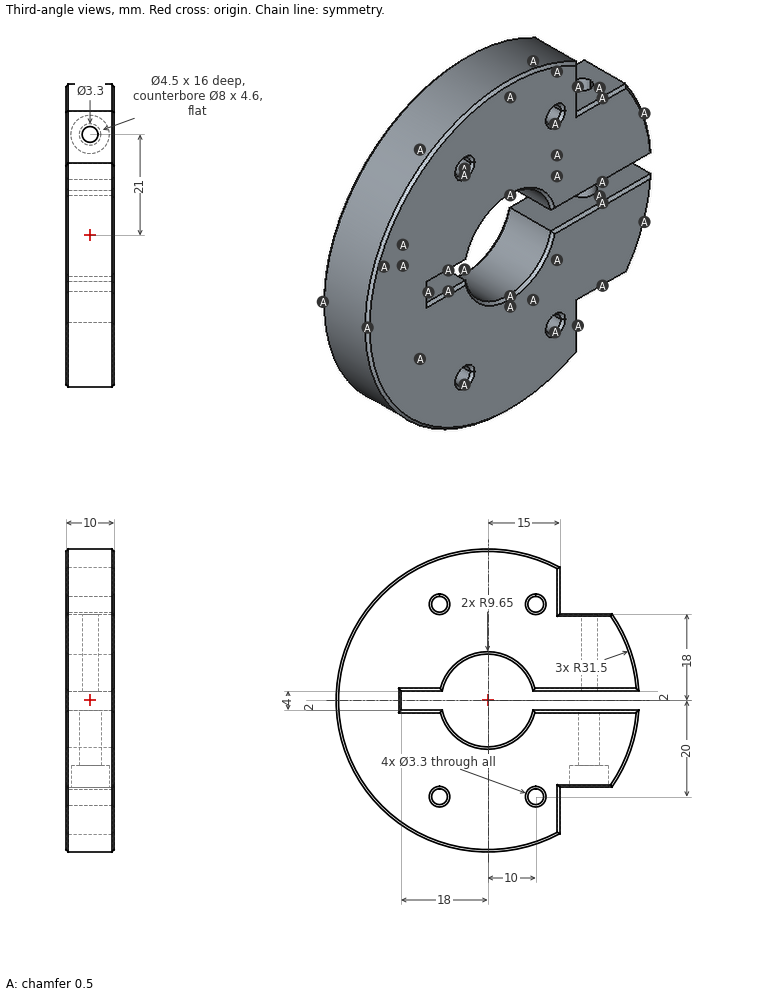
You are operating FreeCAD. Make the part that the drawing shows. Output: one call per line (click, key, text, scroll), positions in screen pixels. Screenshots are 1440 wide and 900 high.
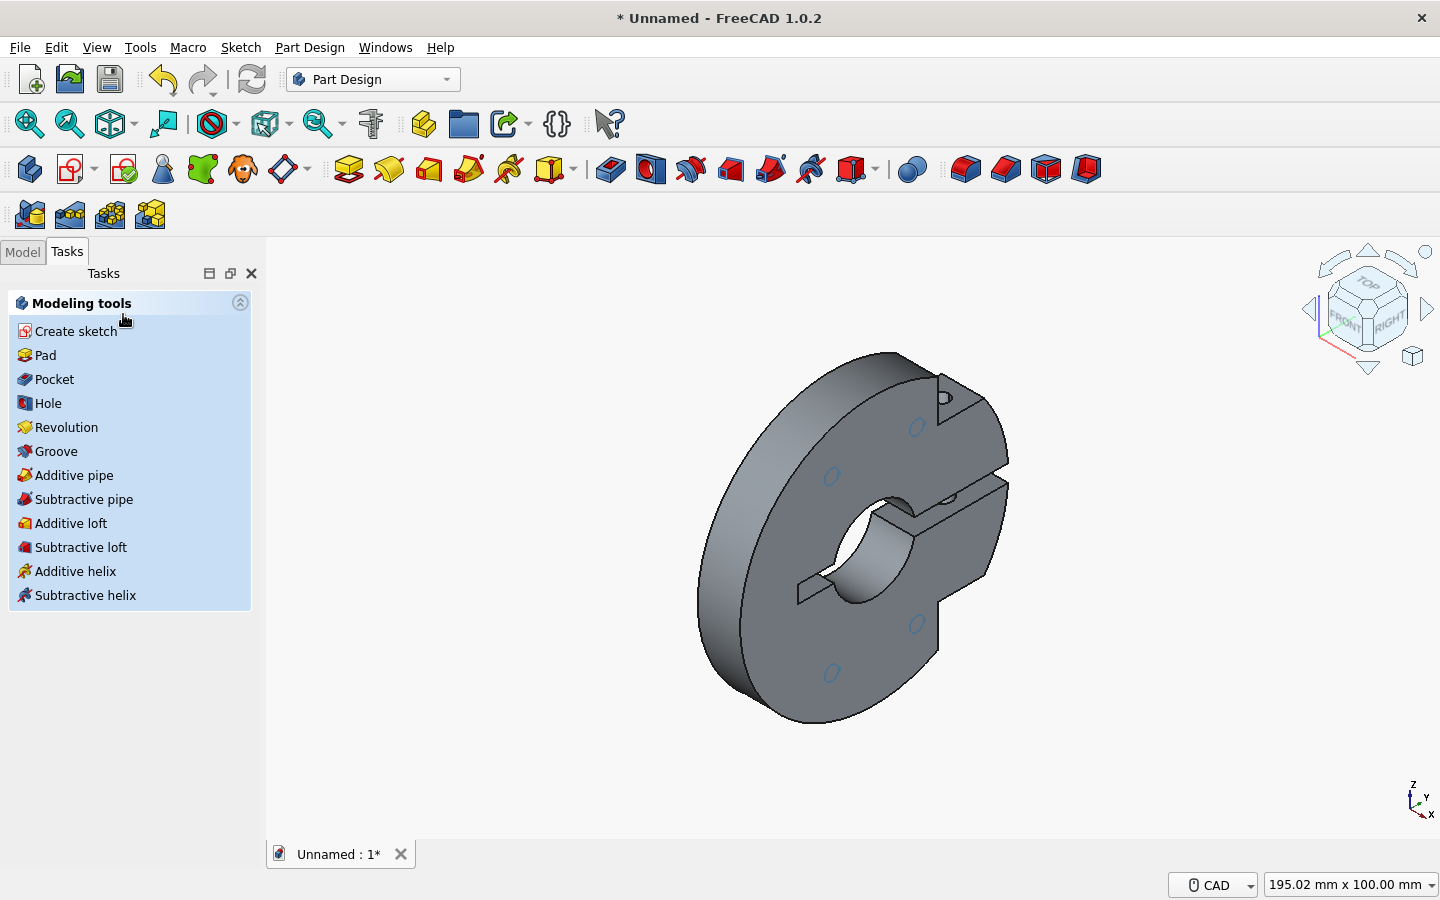
click(652, 170)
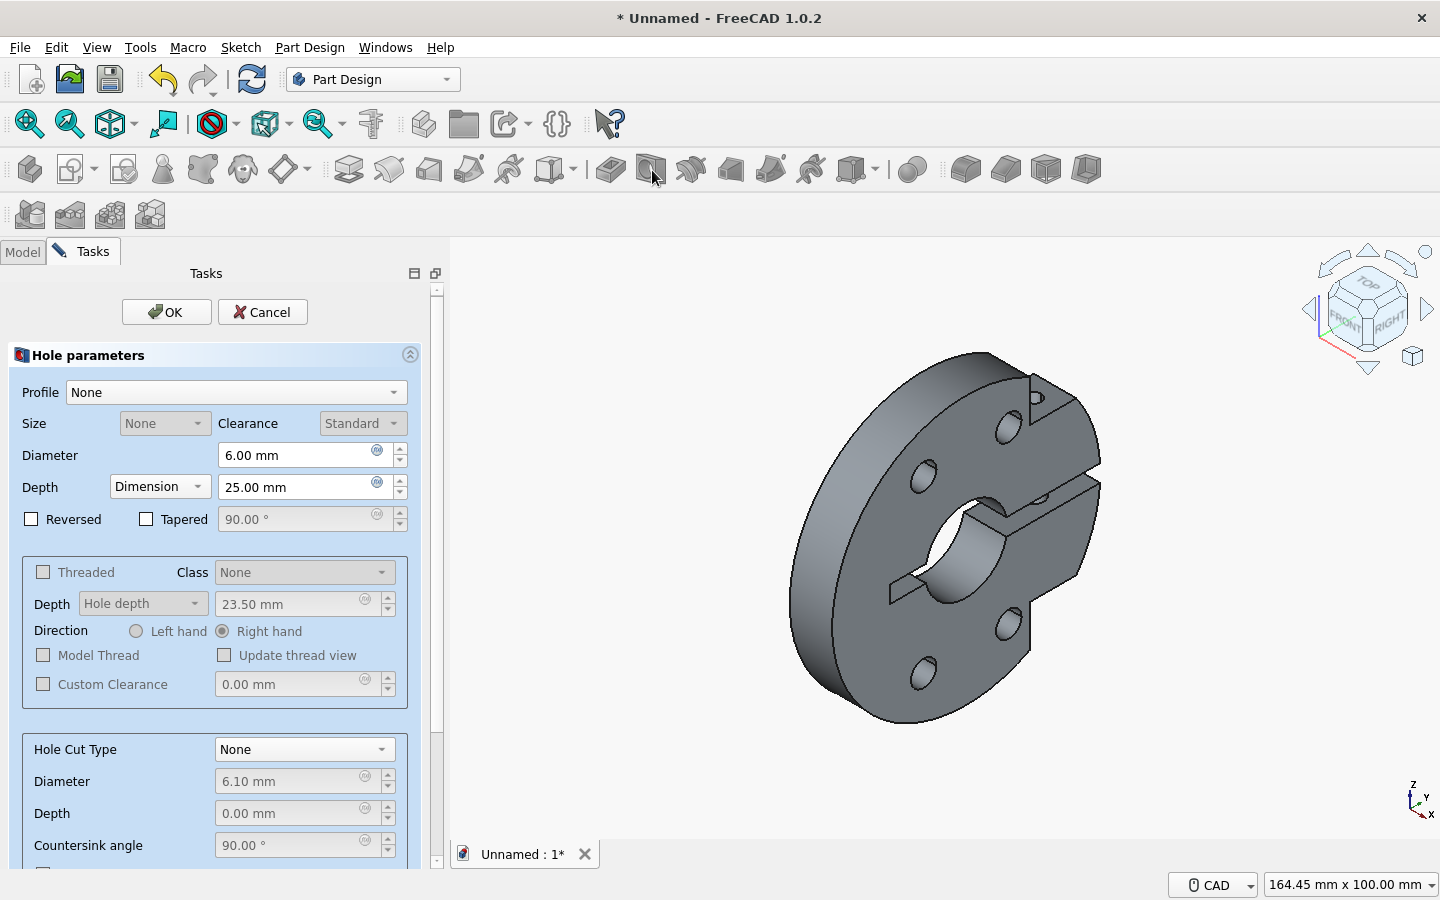
triple_click(305, 455)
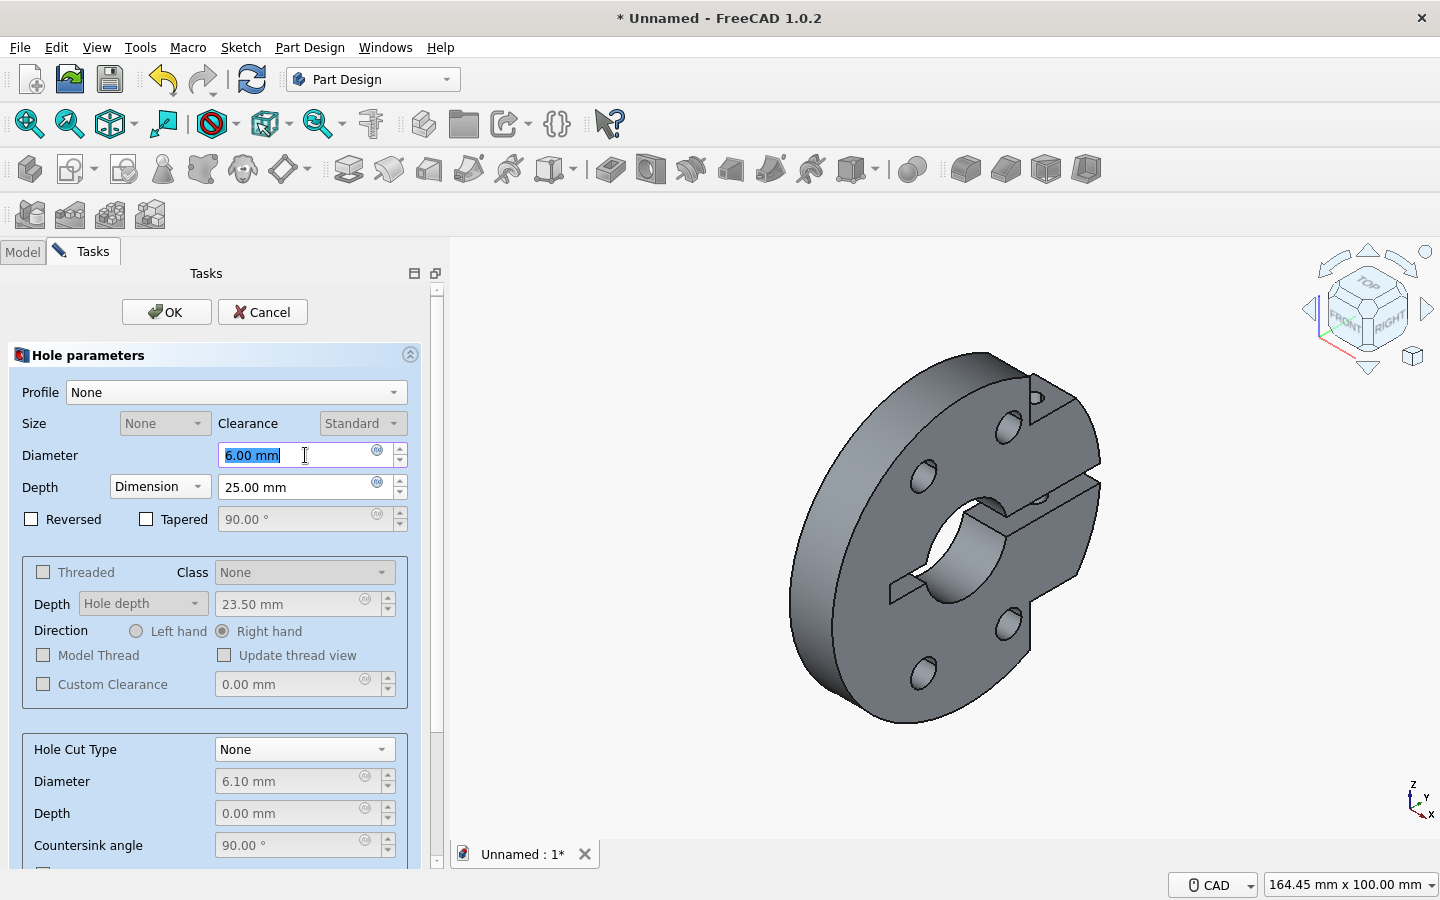
text(3.3)
key(Tab)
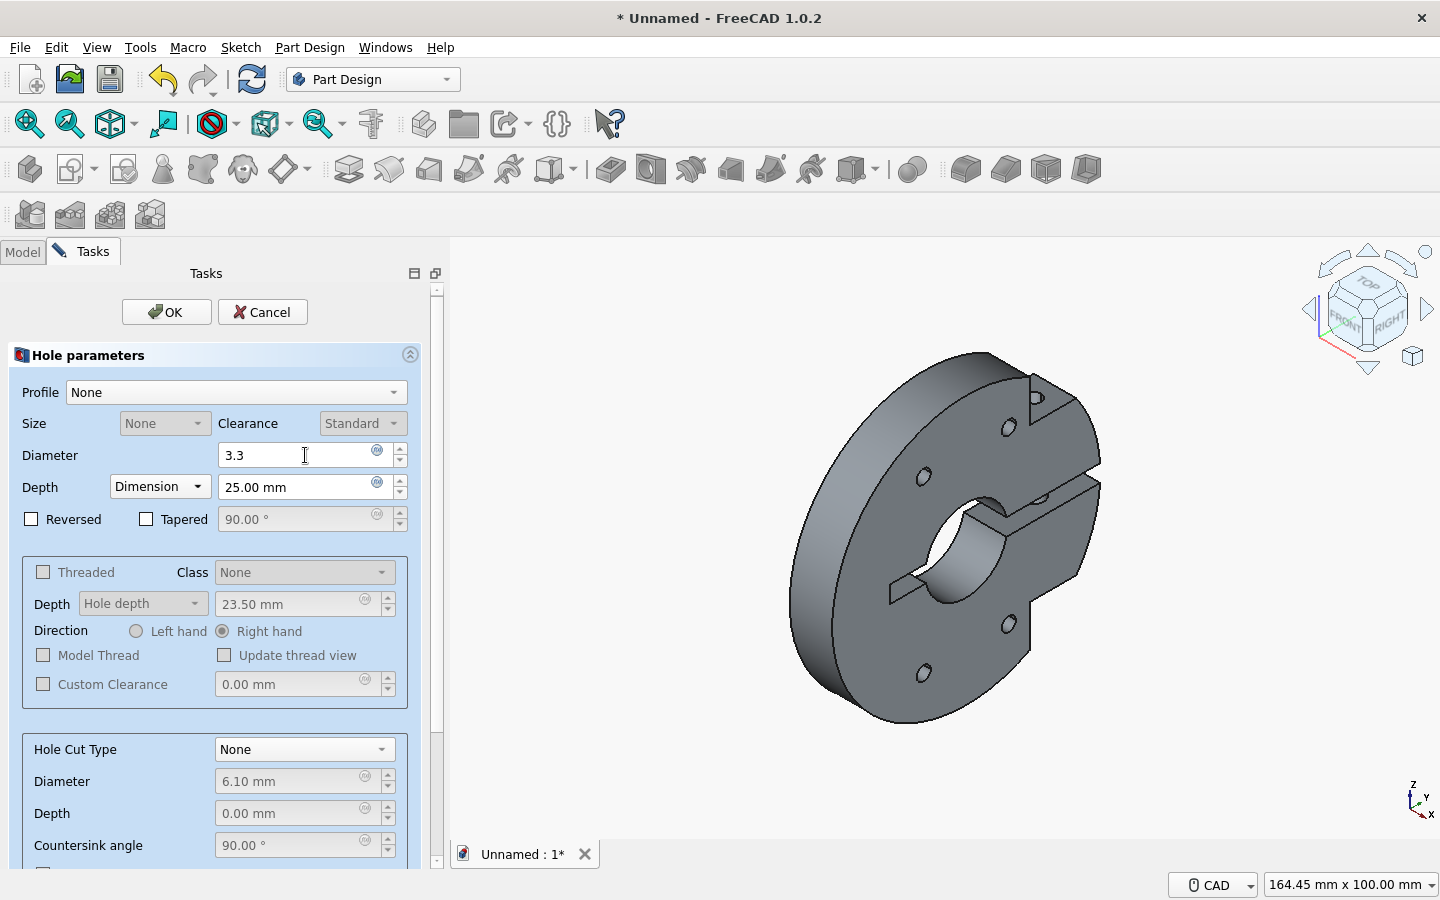
click(161, 486)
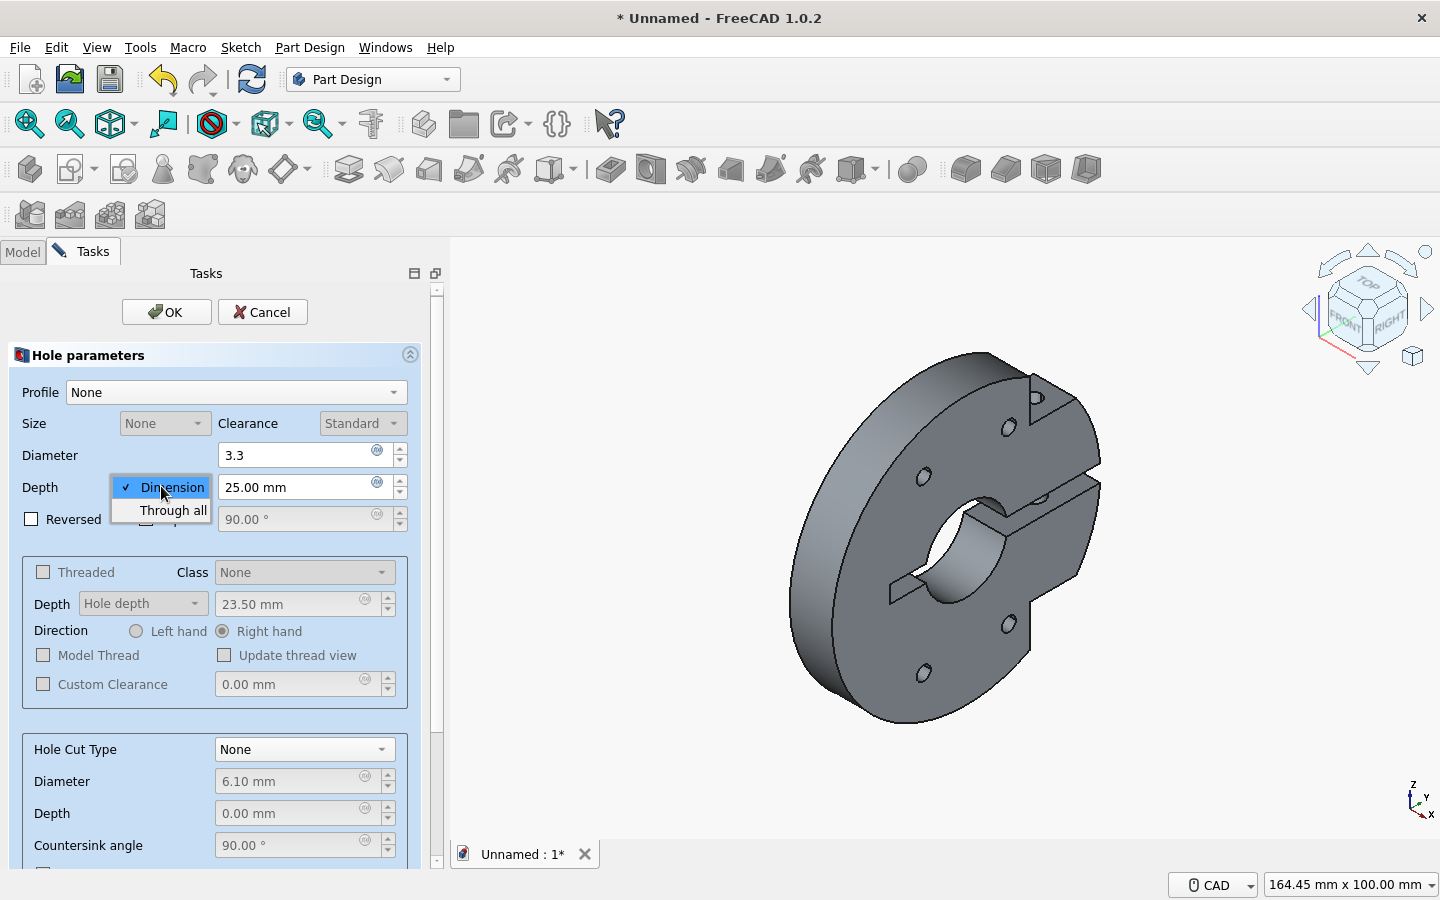
click(160, 510)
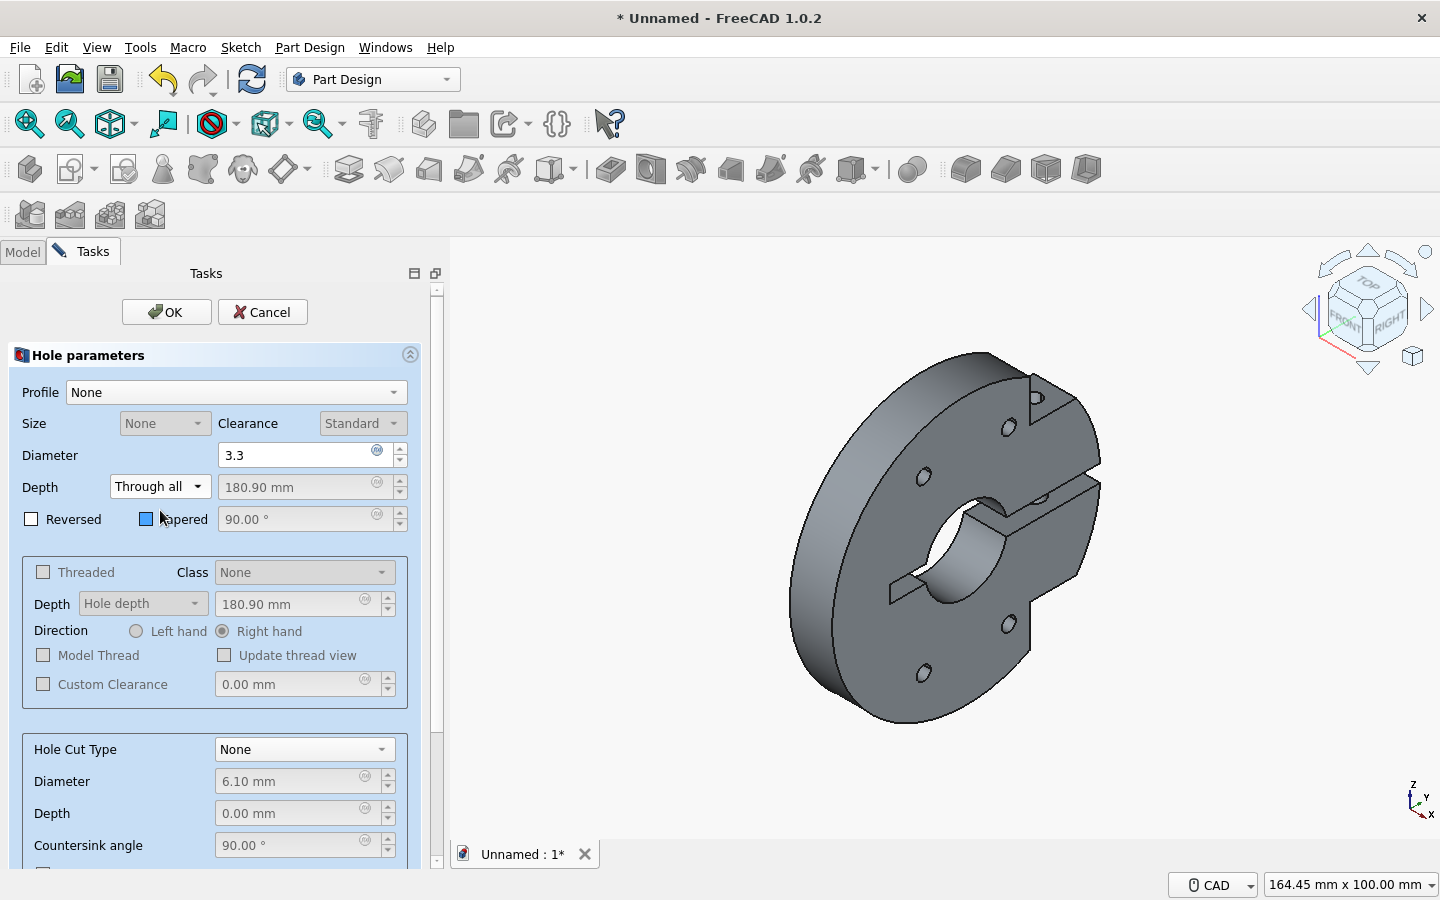
click(167, 312)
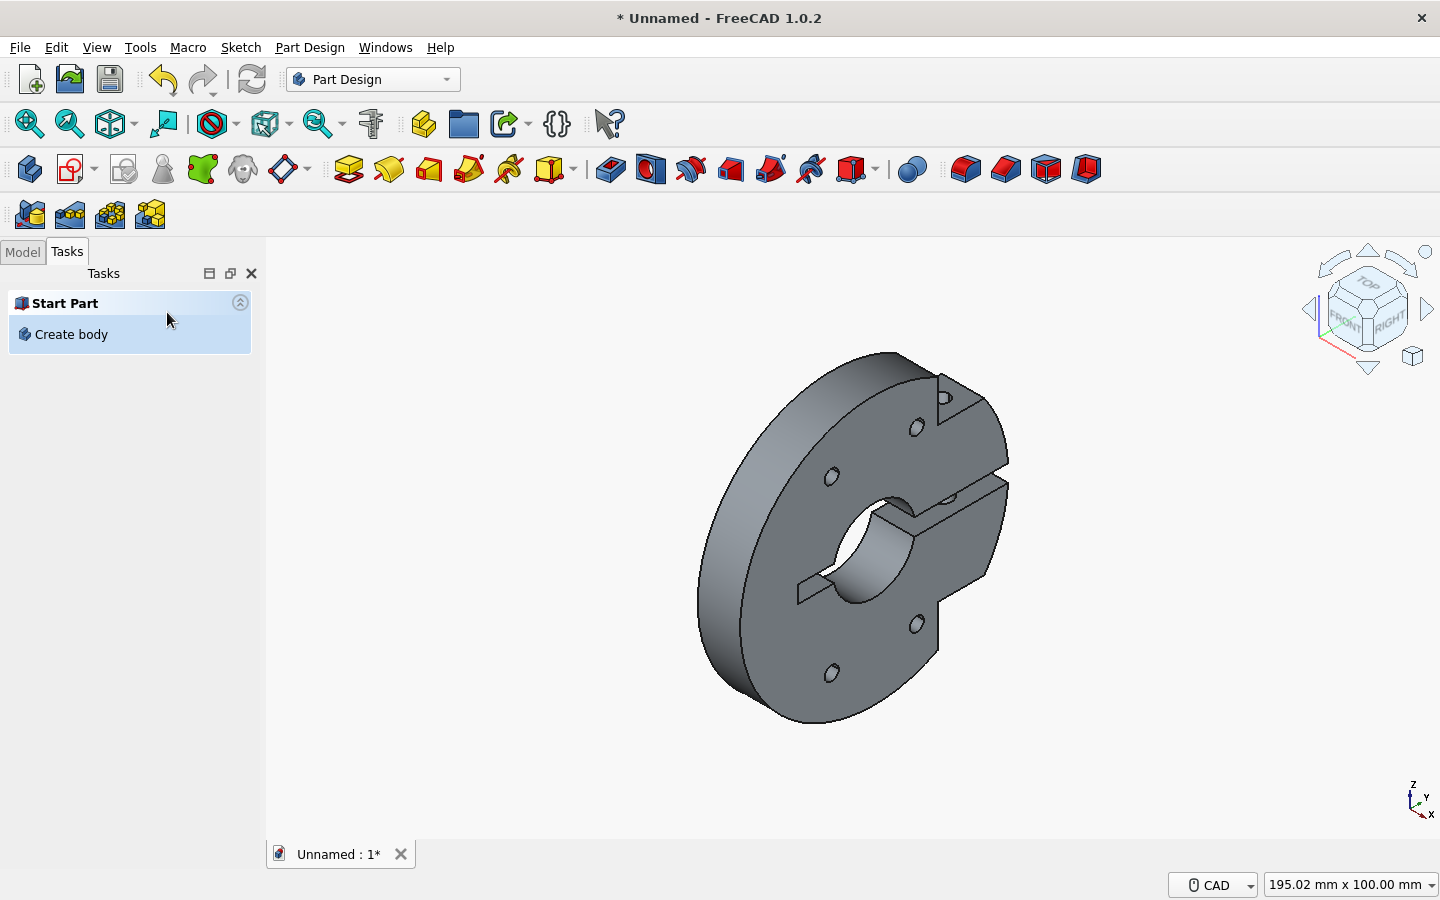
click(874, 461)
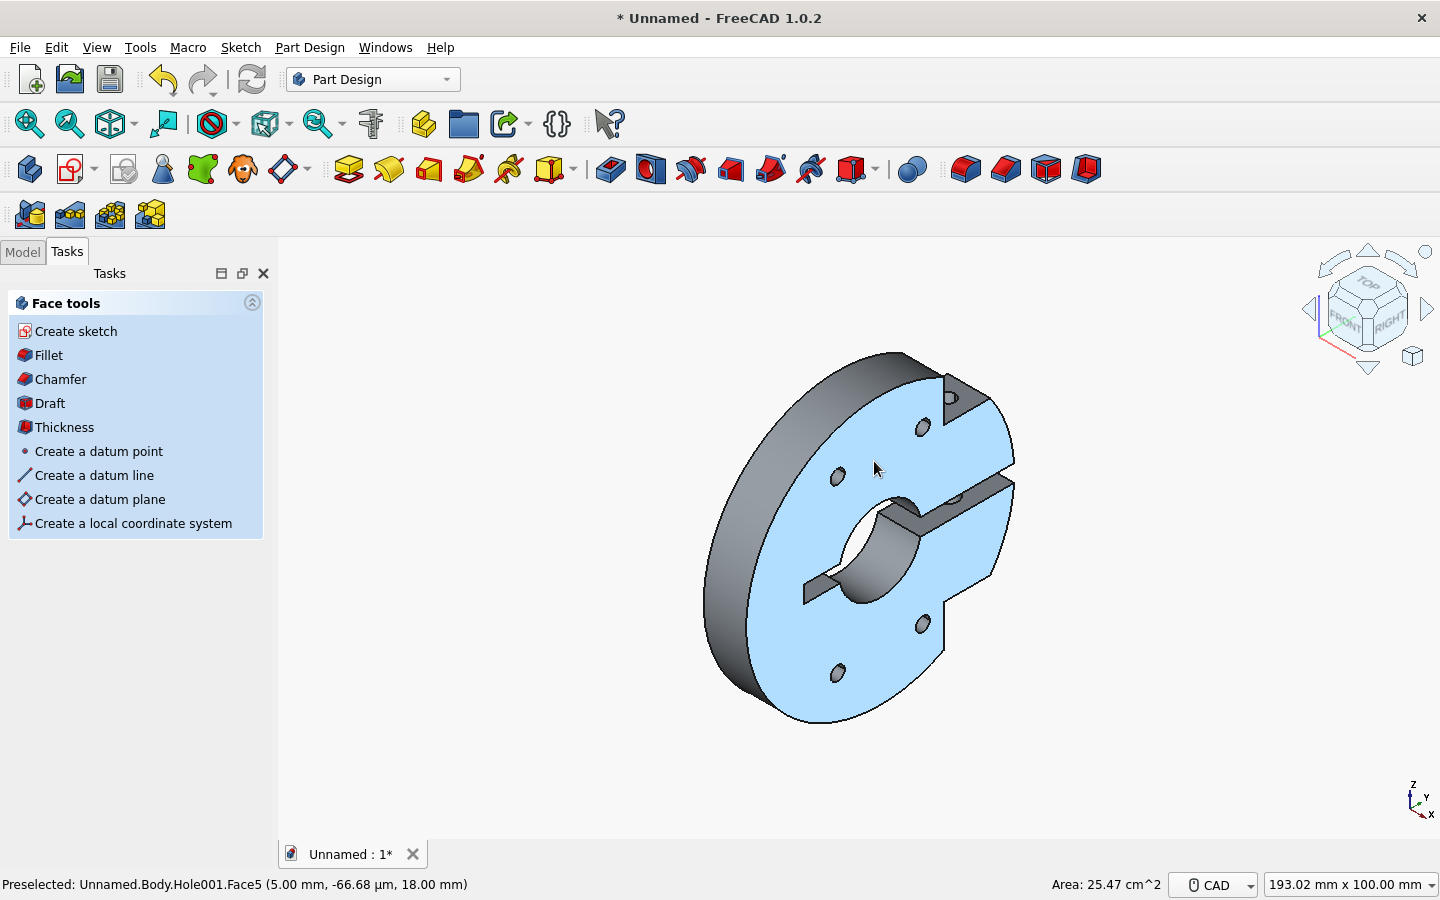
key(2)